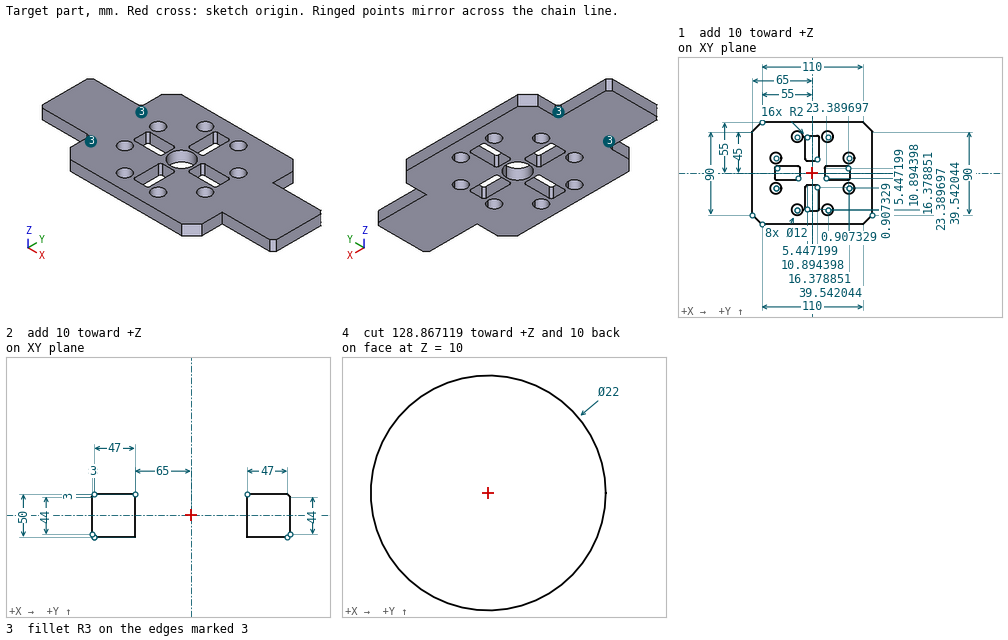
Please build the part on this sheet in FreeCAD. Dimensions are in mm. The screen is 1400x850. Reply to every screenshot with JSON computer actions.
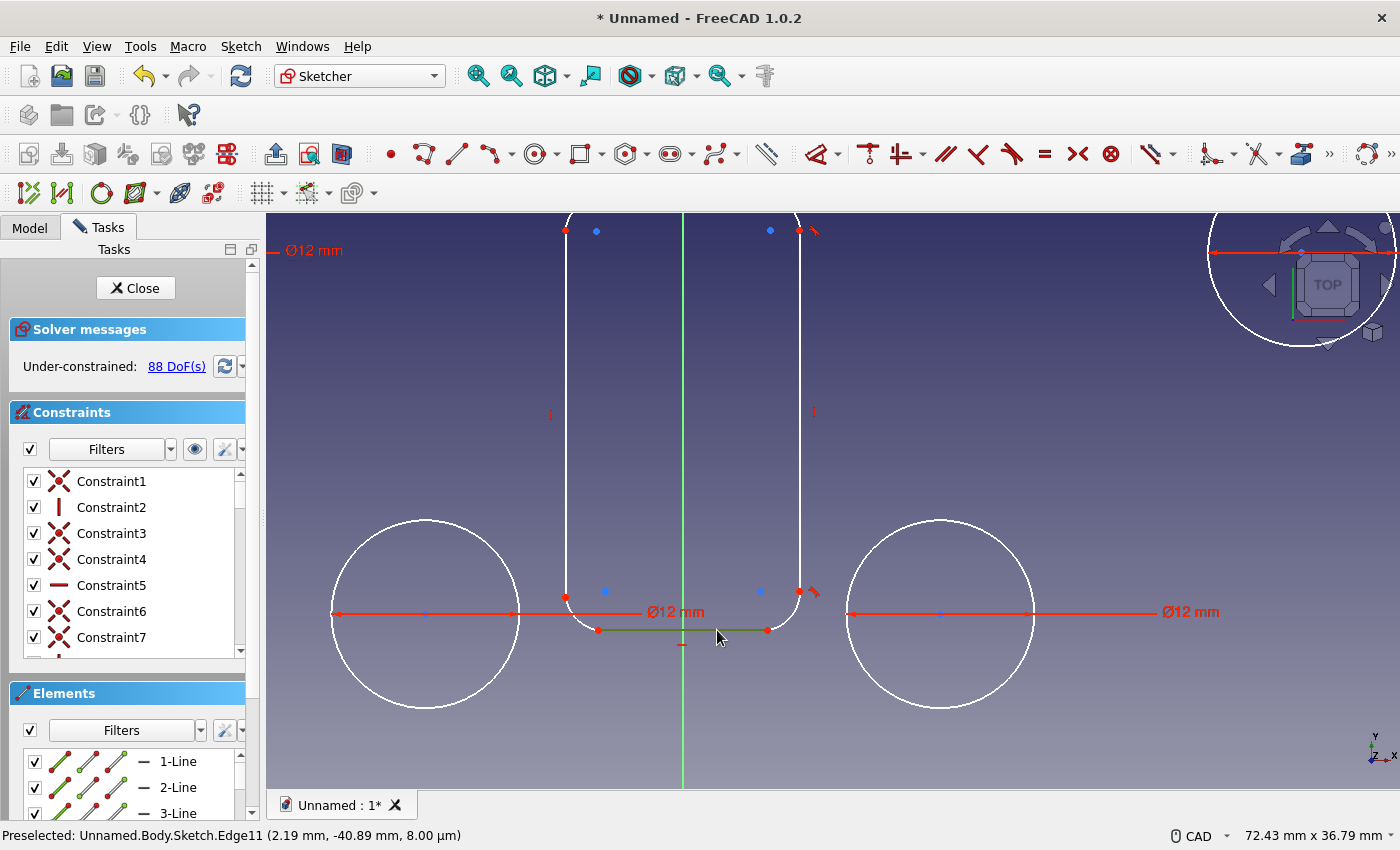
{"action": "left_click", "coordinate": [782, 624]}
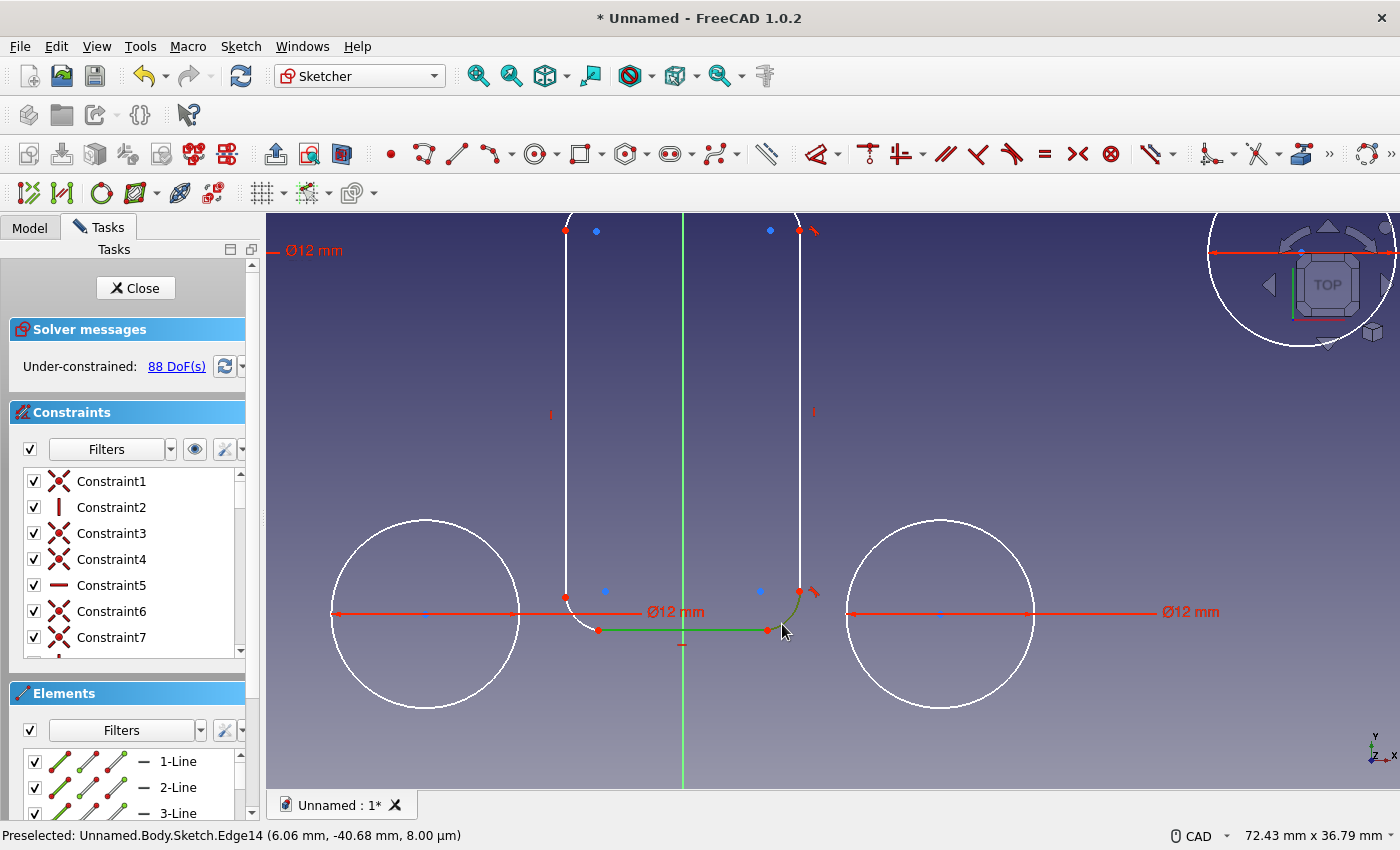
{"action": "left_click", "coordinate": [1012, 154]}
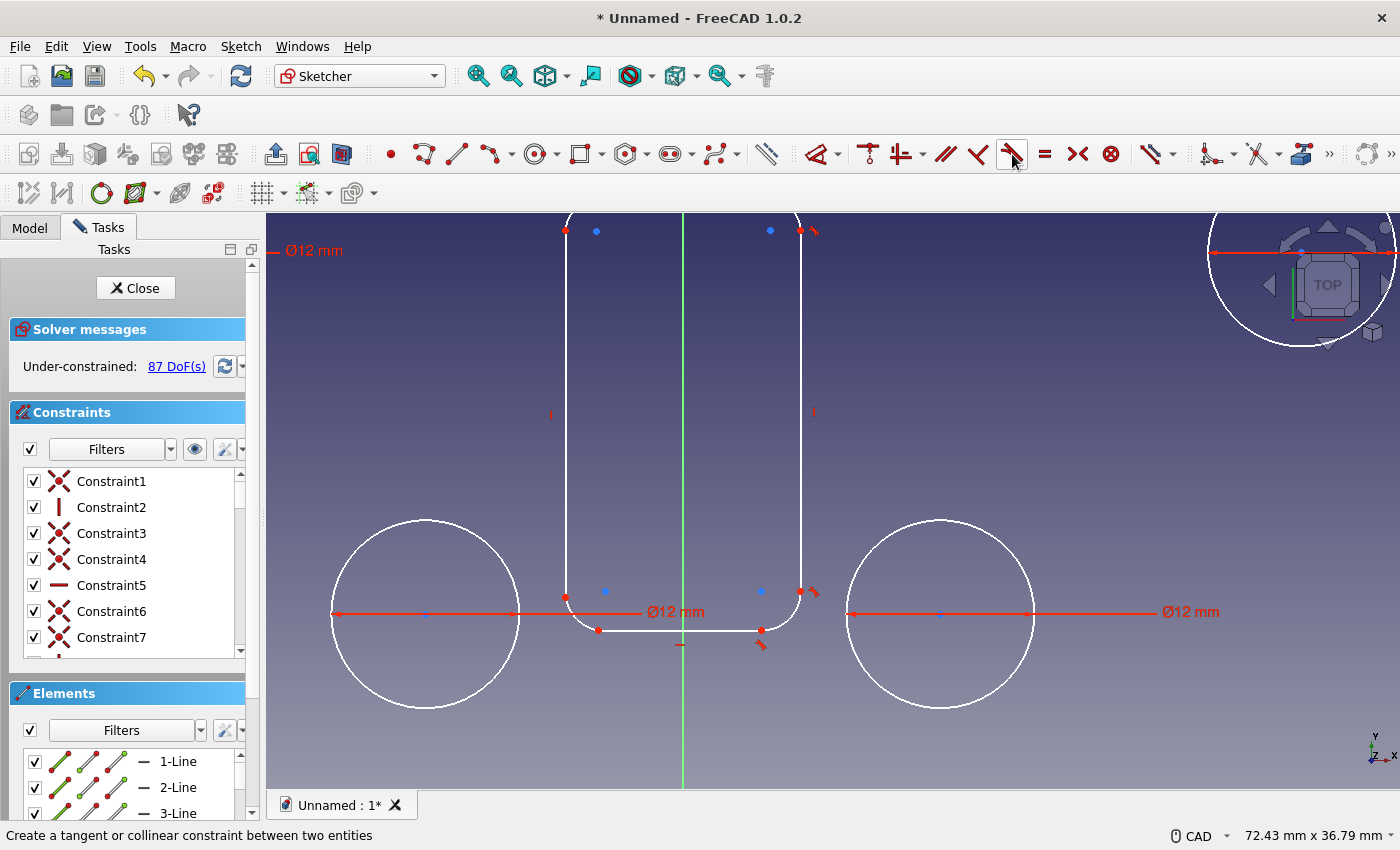
{"action": "left_click", "coordinate": [713, 631]}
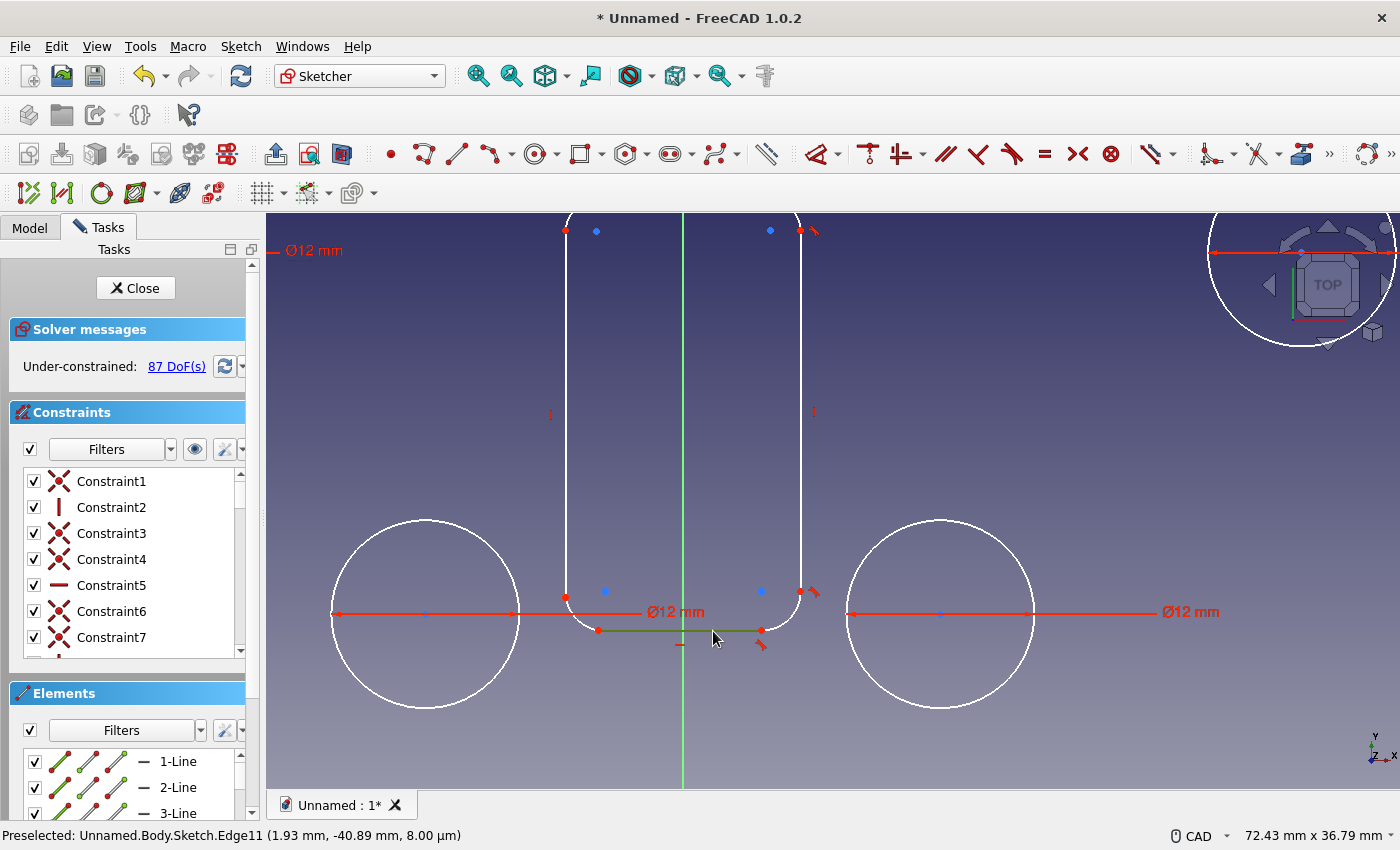
{"action": "left_click", "coordinate": [571, 612]}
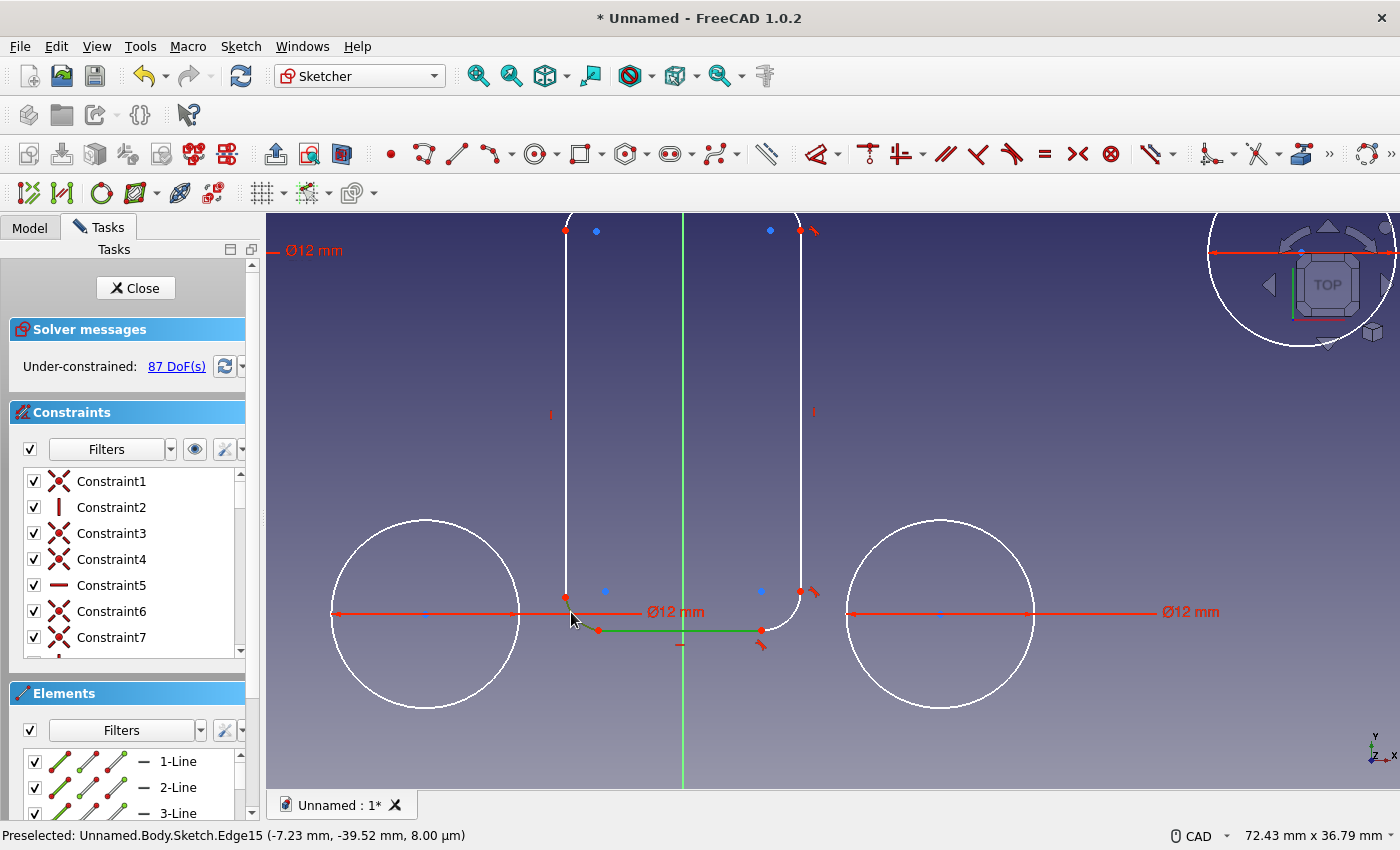
{"action": "left_click", "coordinate": [1012, 154]}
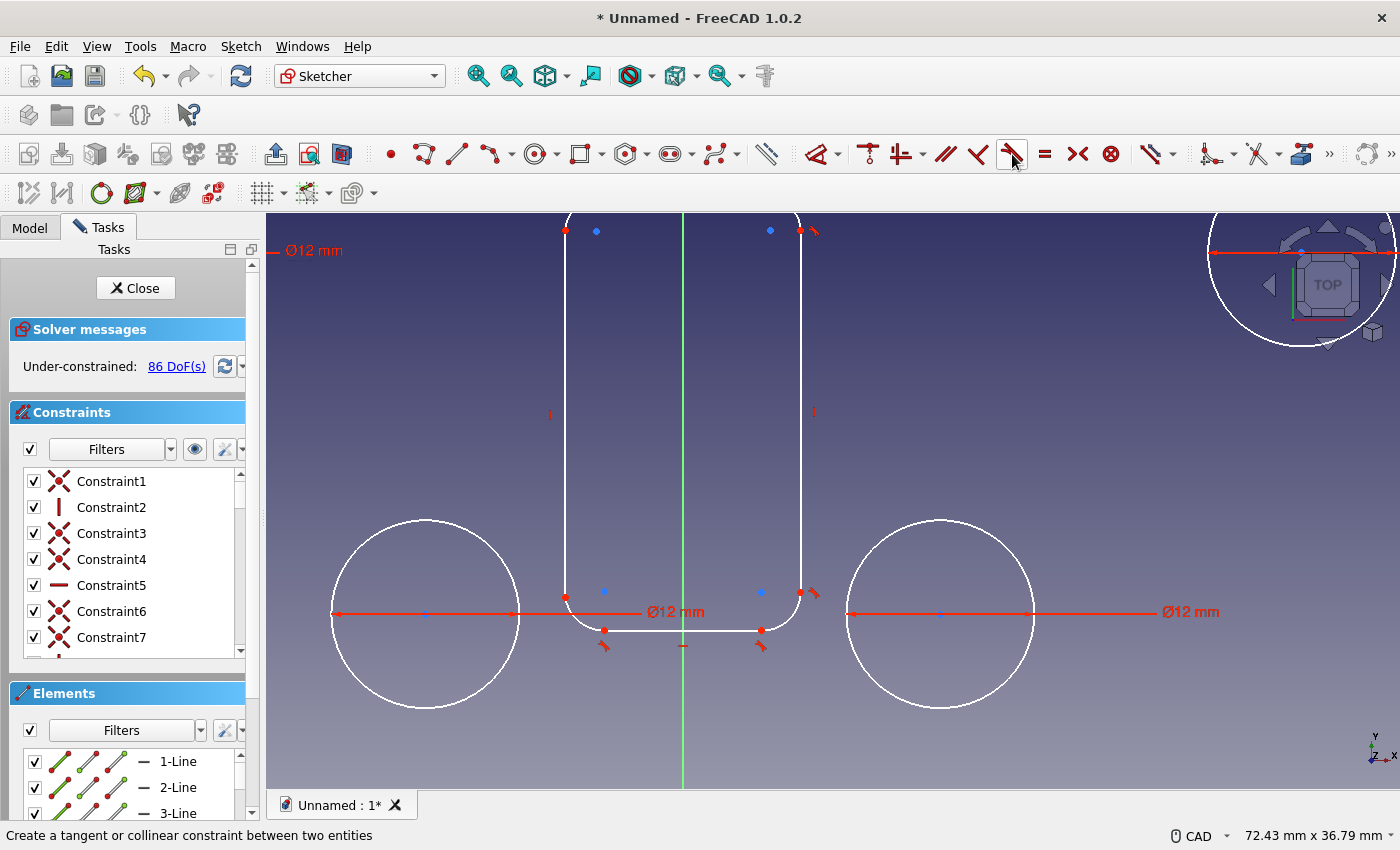
{"action": "scroll", "coordinate": [785, 630], "scroll_direction": "down", "scroll_amount": 8}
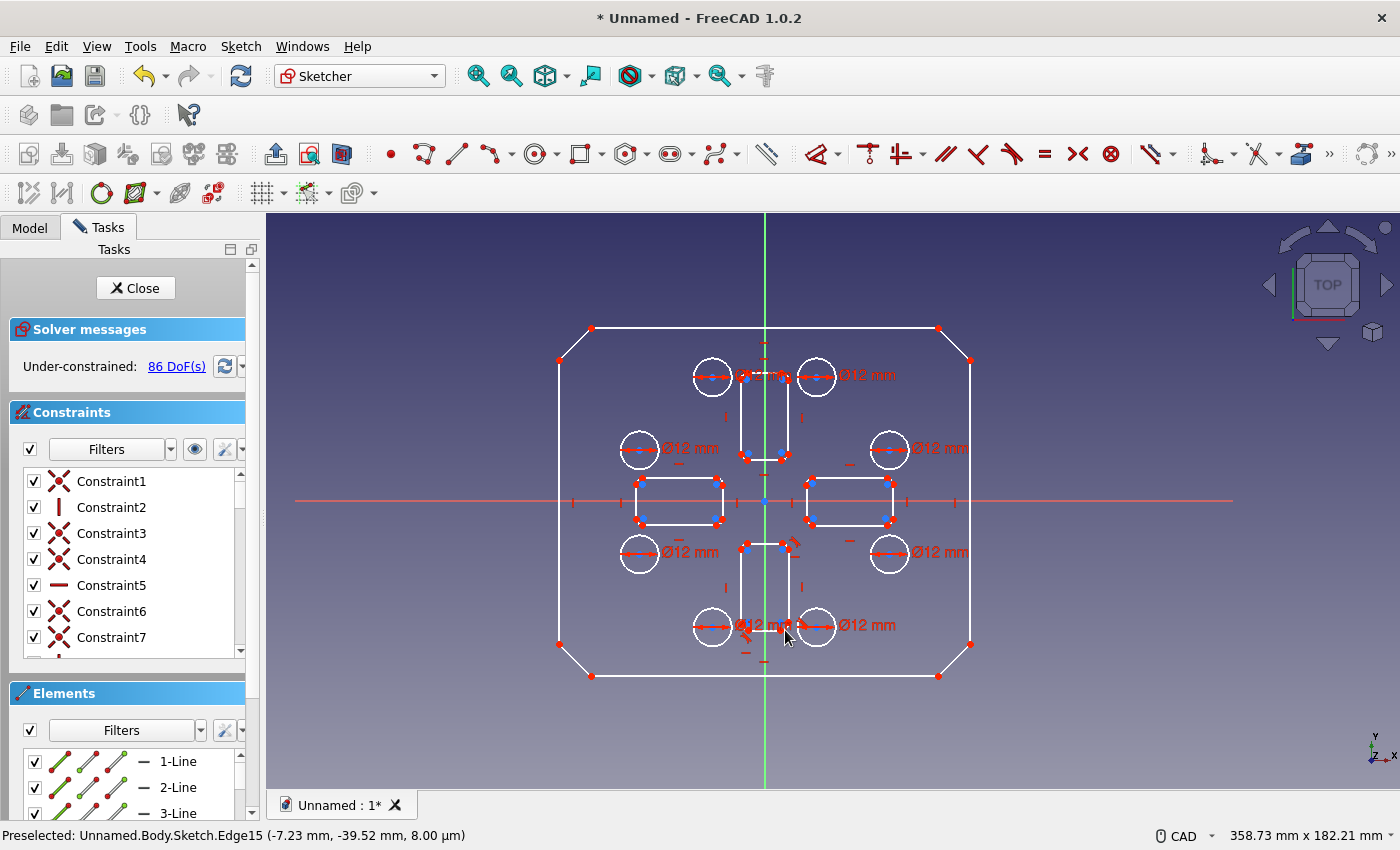
{"action": "left_click", "coordinate": [741, 602]}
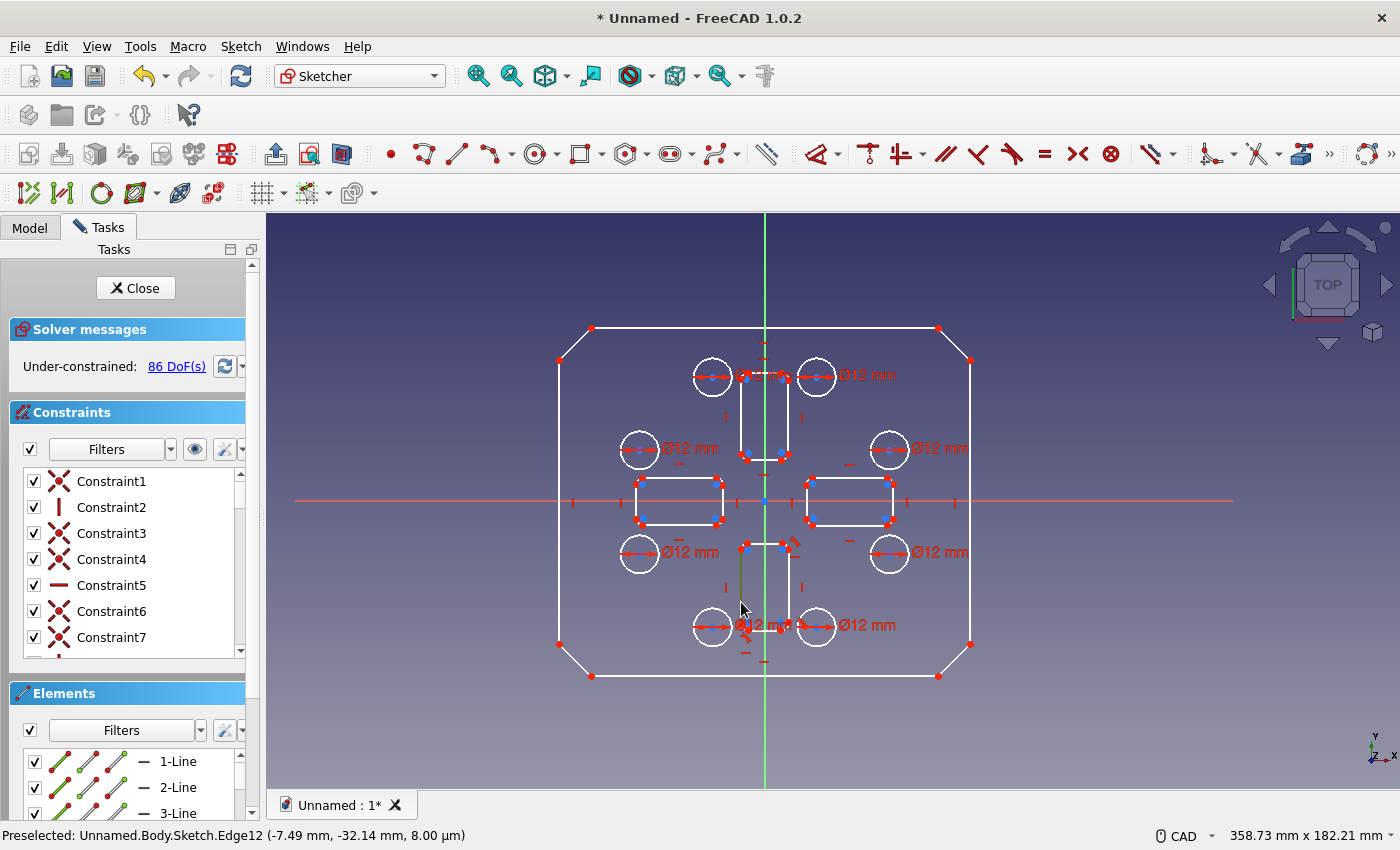
{"action": "scroll", "coordinate": [744, 629], "scroll_direction": "up", "scroll_amount": 5}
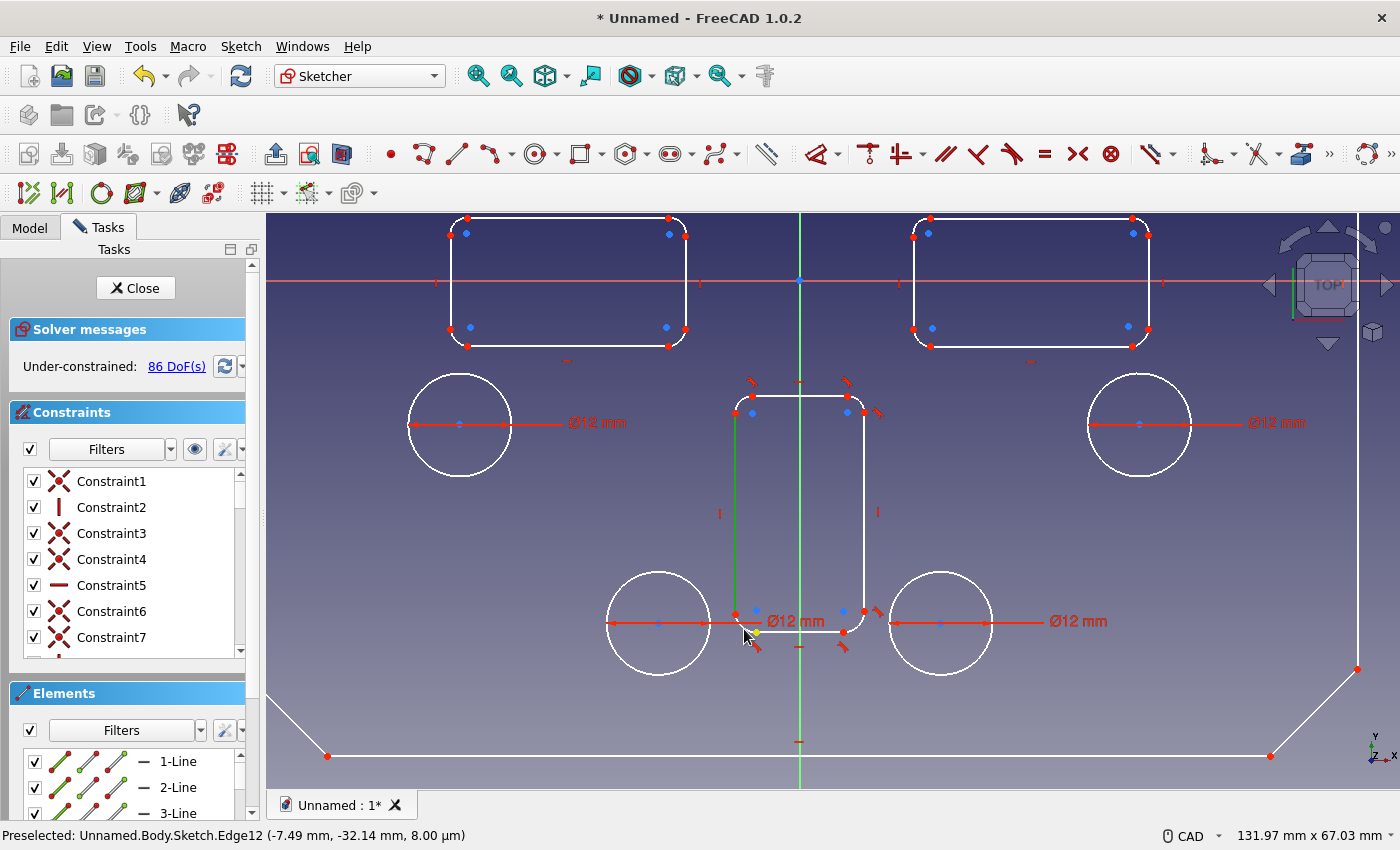
{"action": "left_click", "coordinate": [743, 627]}